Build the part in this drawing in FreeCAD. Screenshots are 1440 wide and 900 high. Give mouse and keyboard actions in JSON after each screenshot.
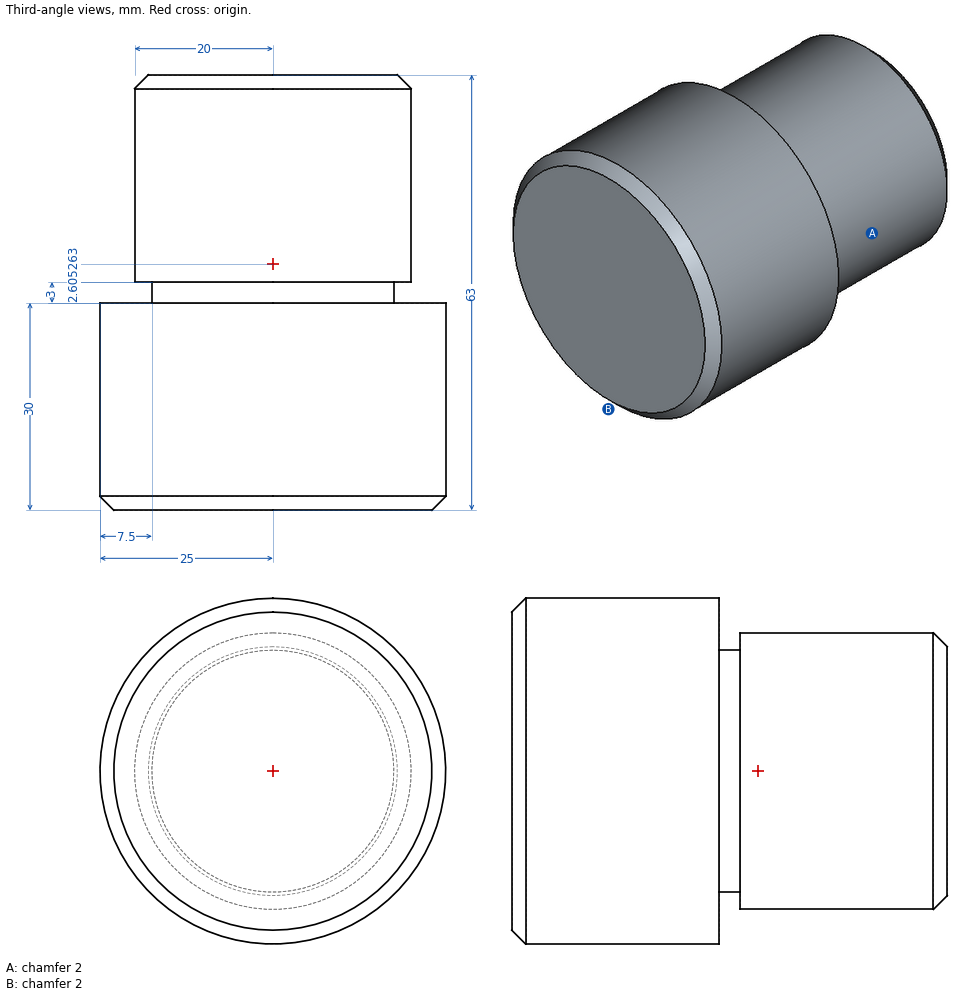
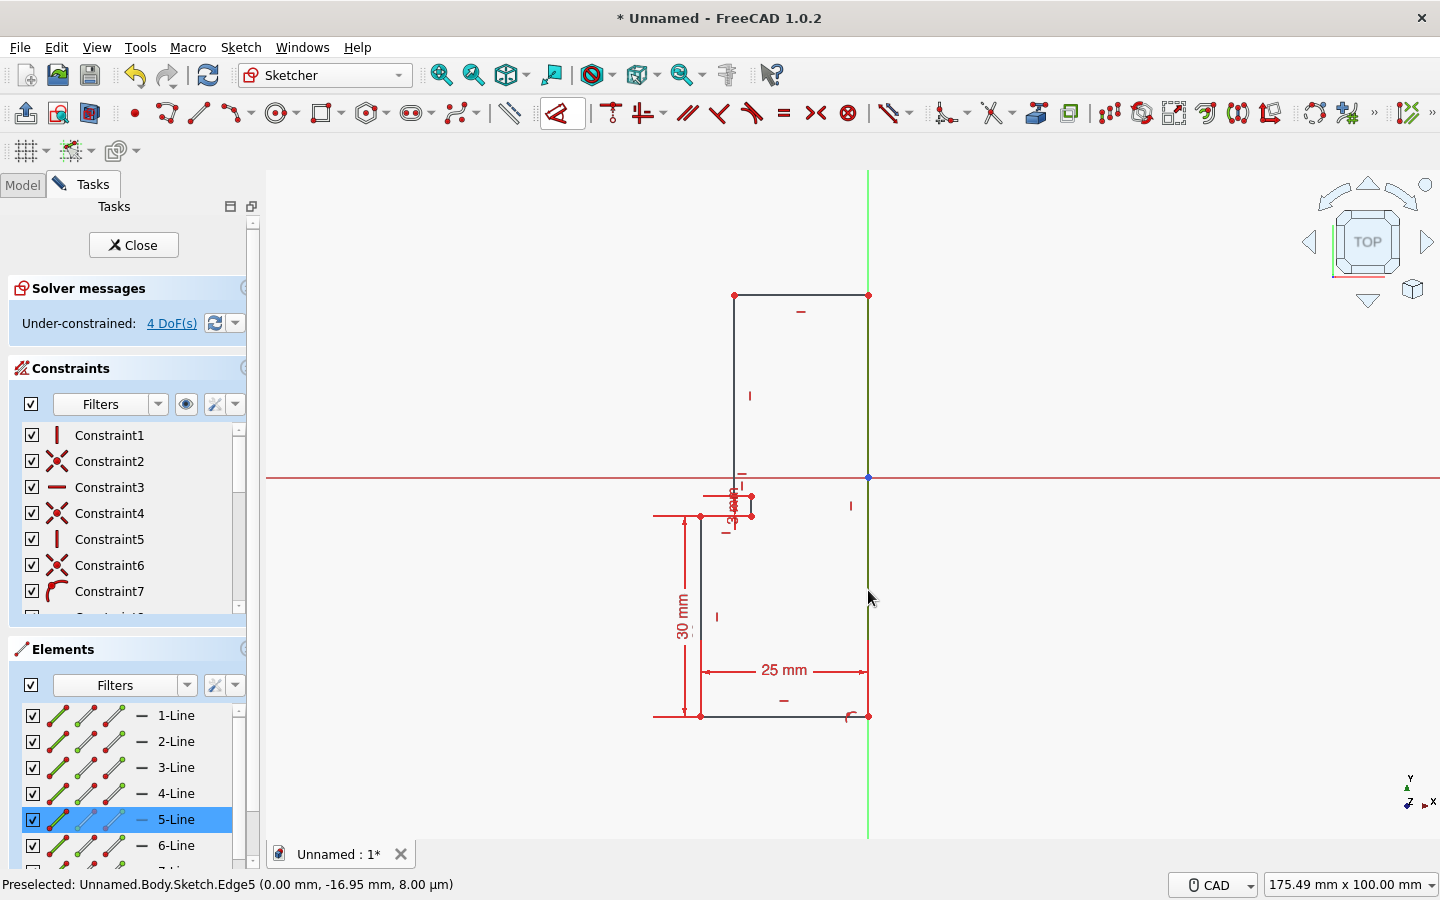
{"action": "left_click", "coordinate": [580, 114]}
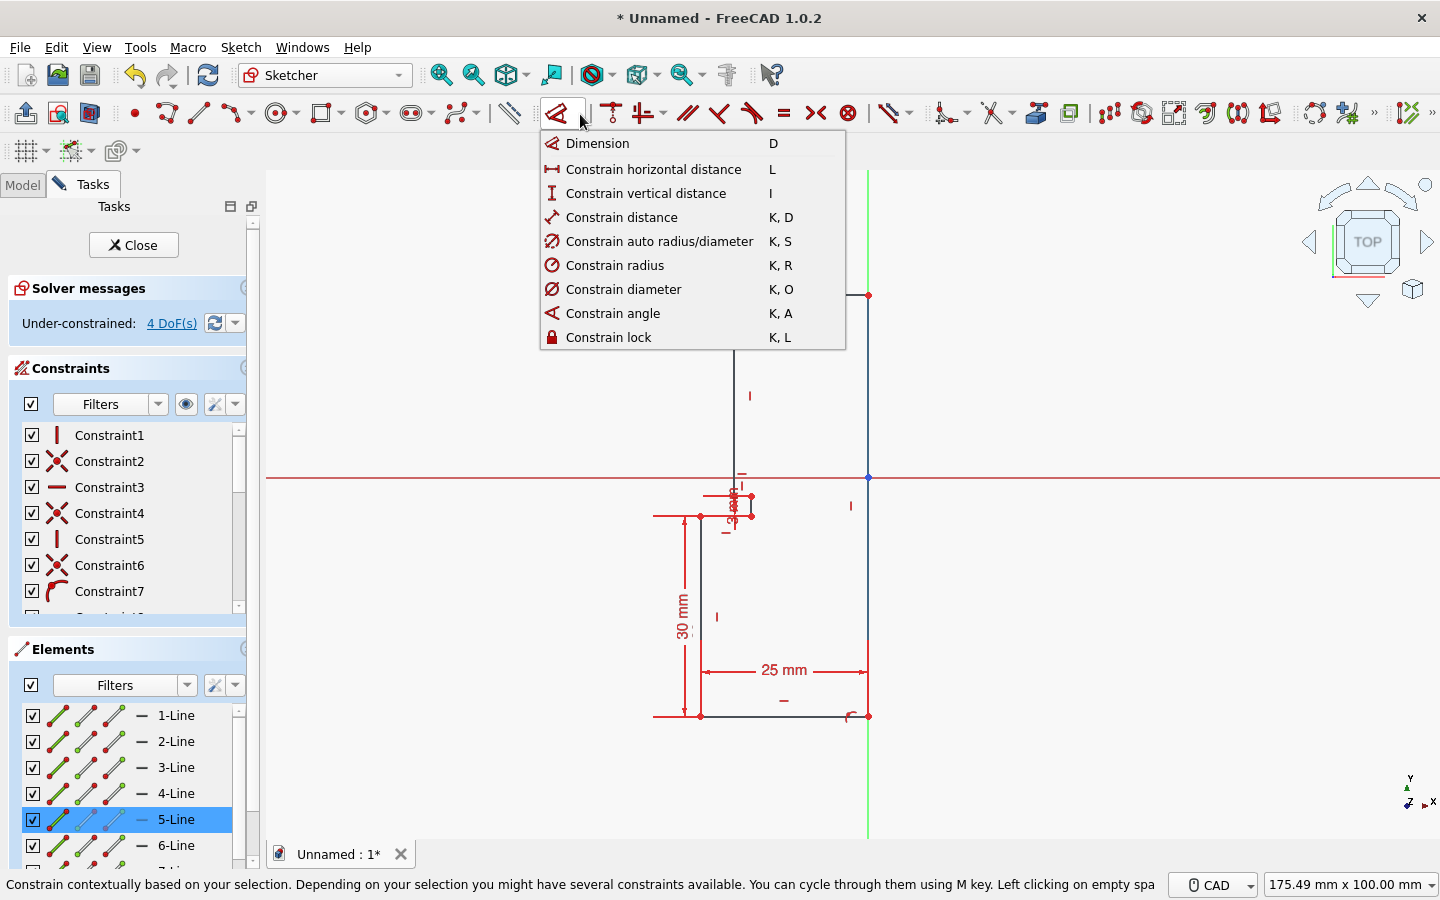
{"action": "left_click", "coordinate": [693, 193]}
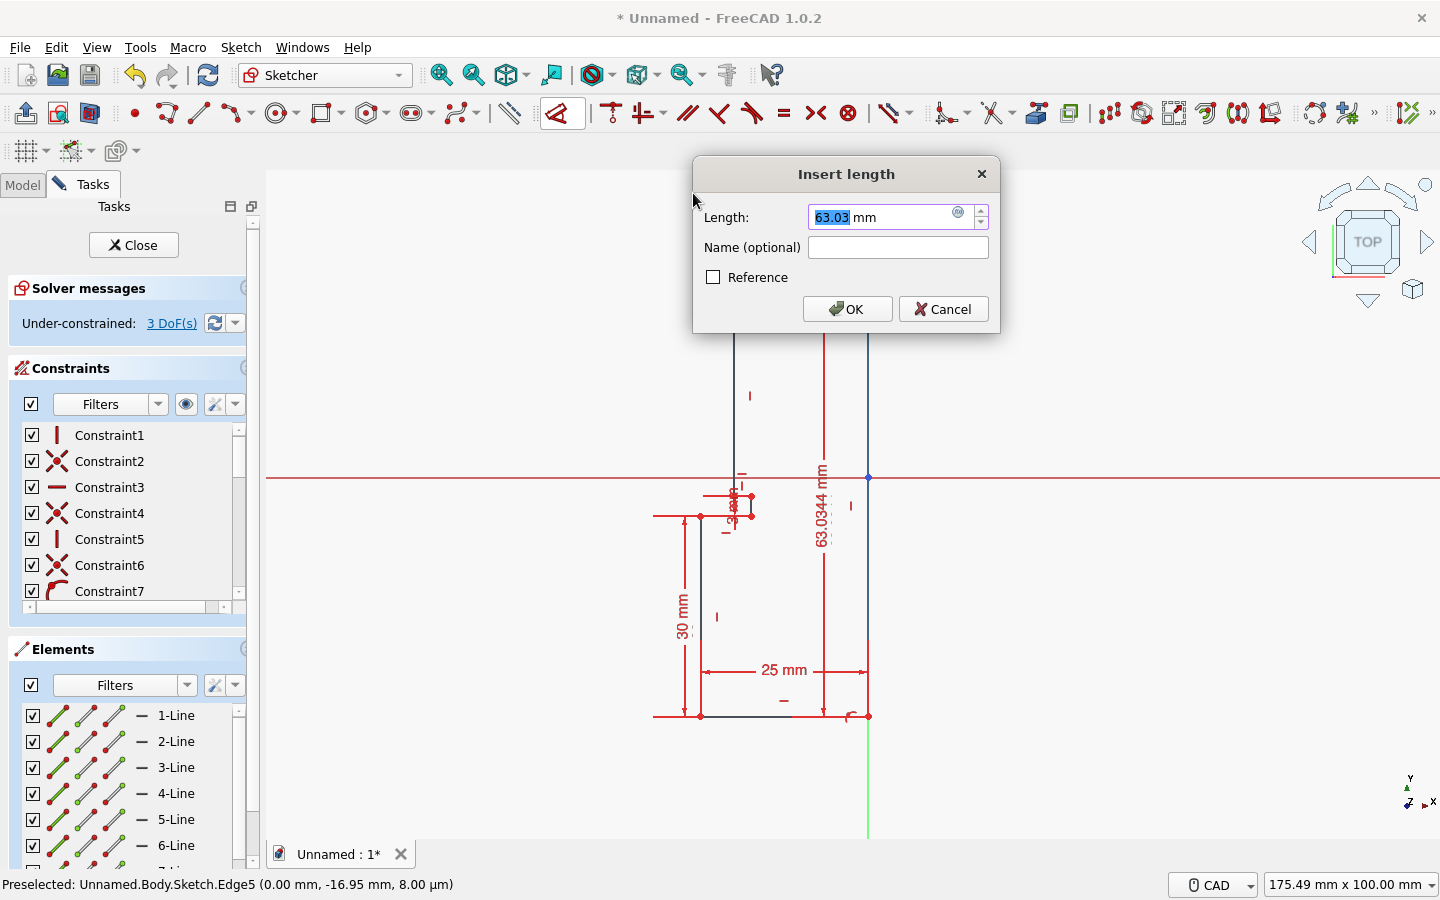
{"action": "type", "text": "63"}
{"action": "key", "text": "Return"}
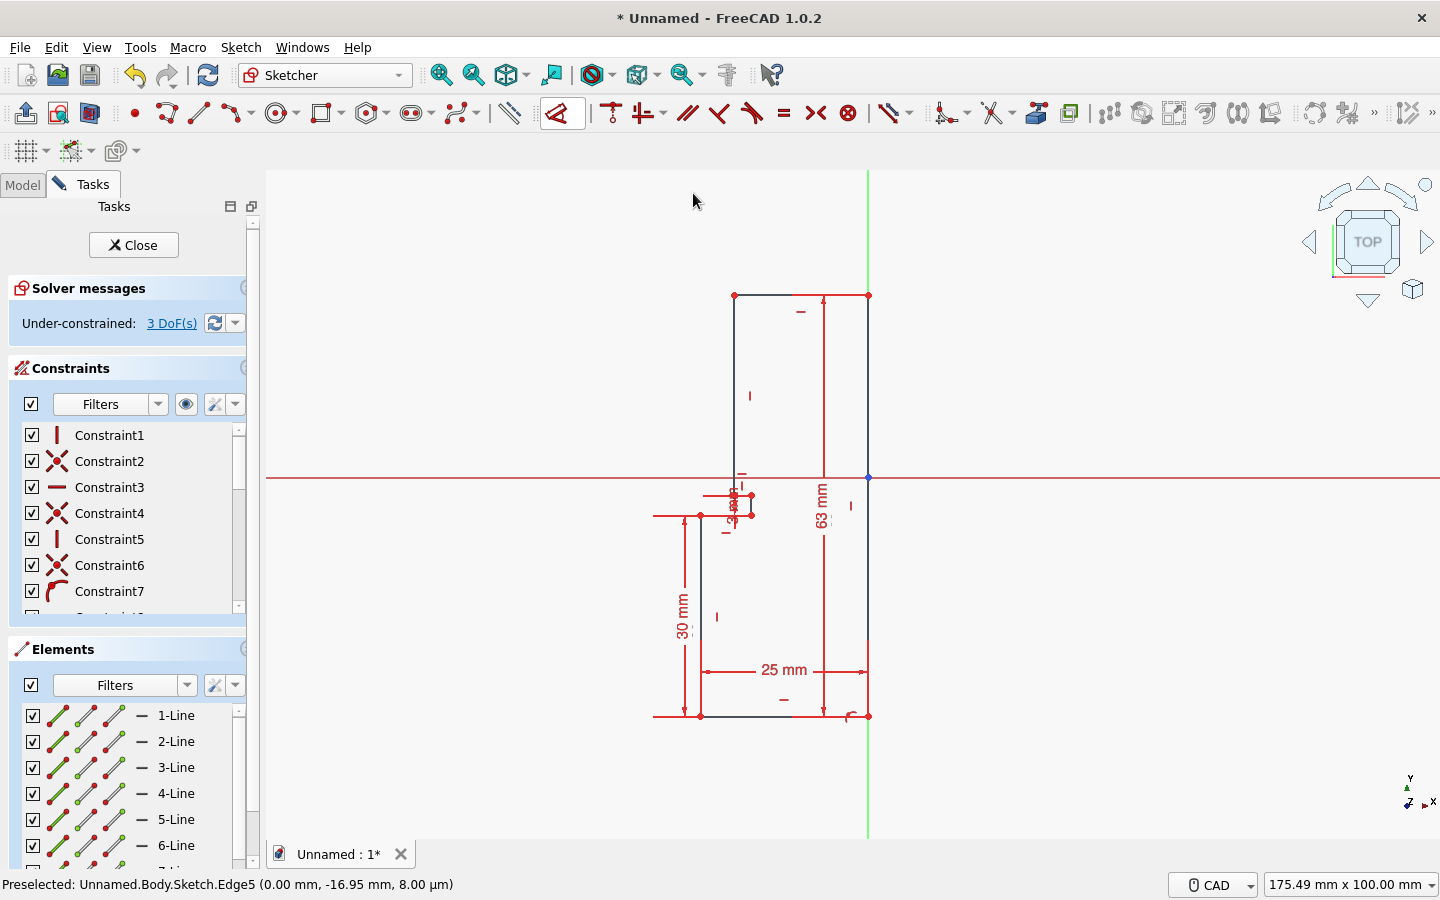
{"action": "left_click", "coordinate": [828, 295]}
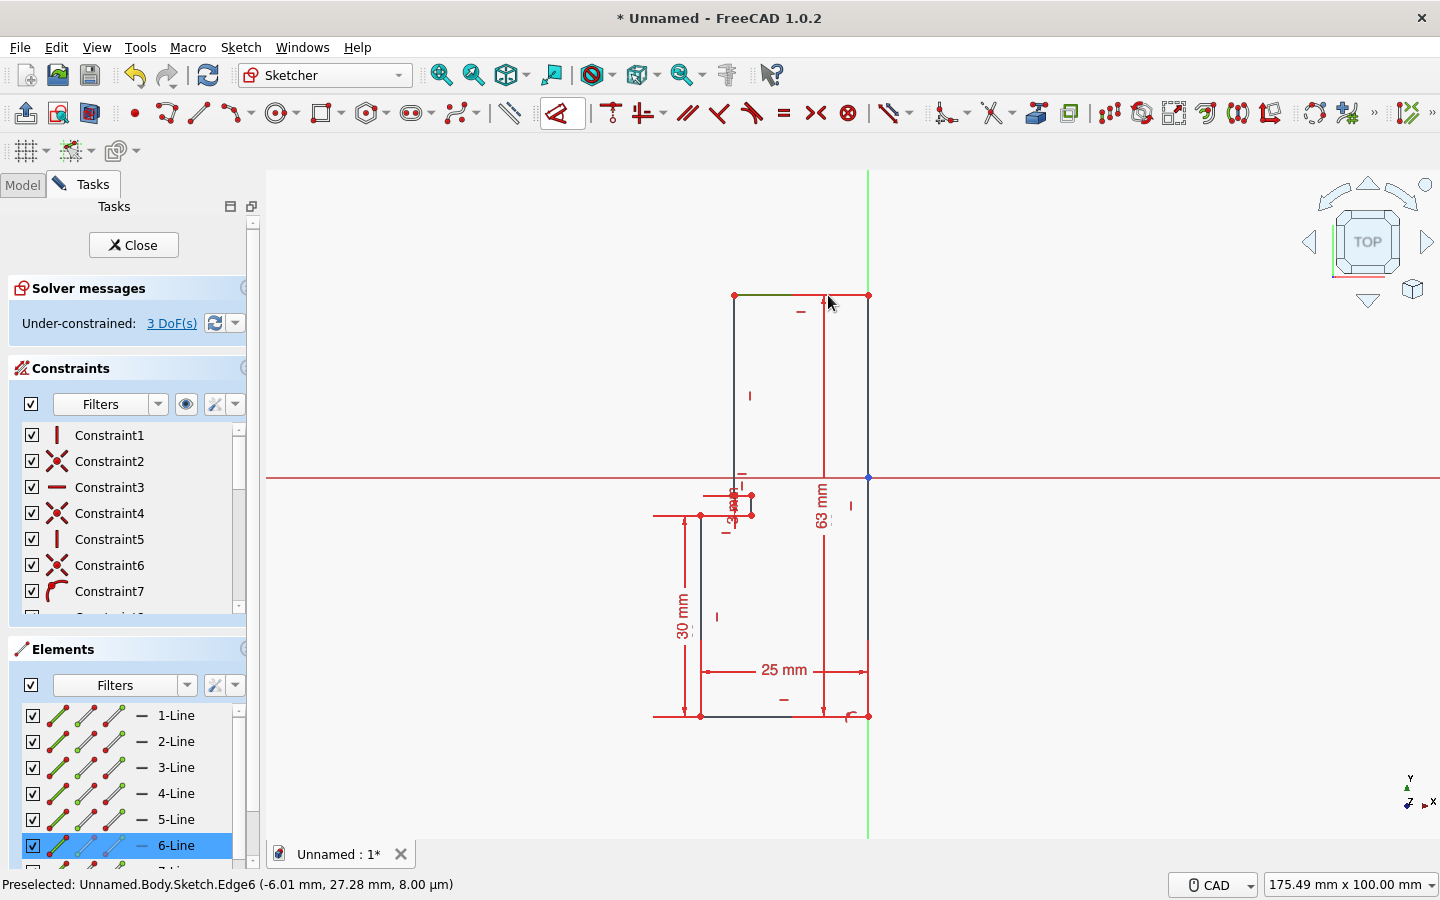
{"action": "left_click", "coordinate": [580, 114]}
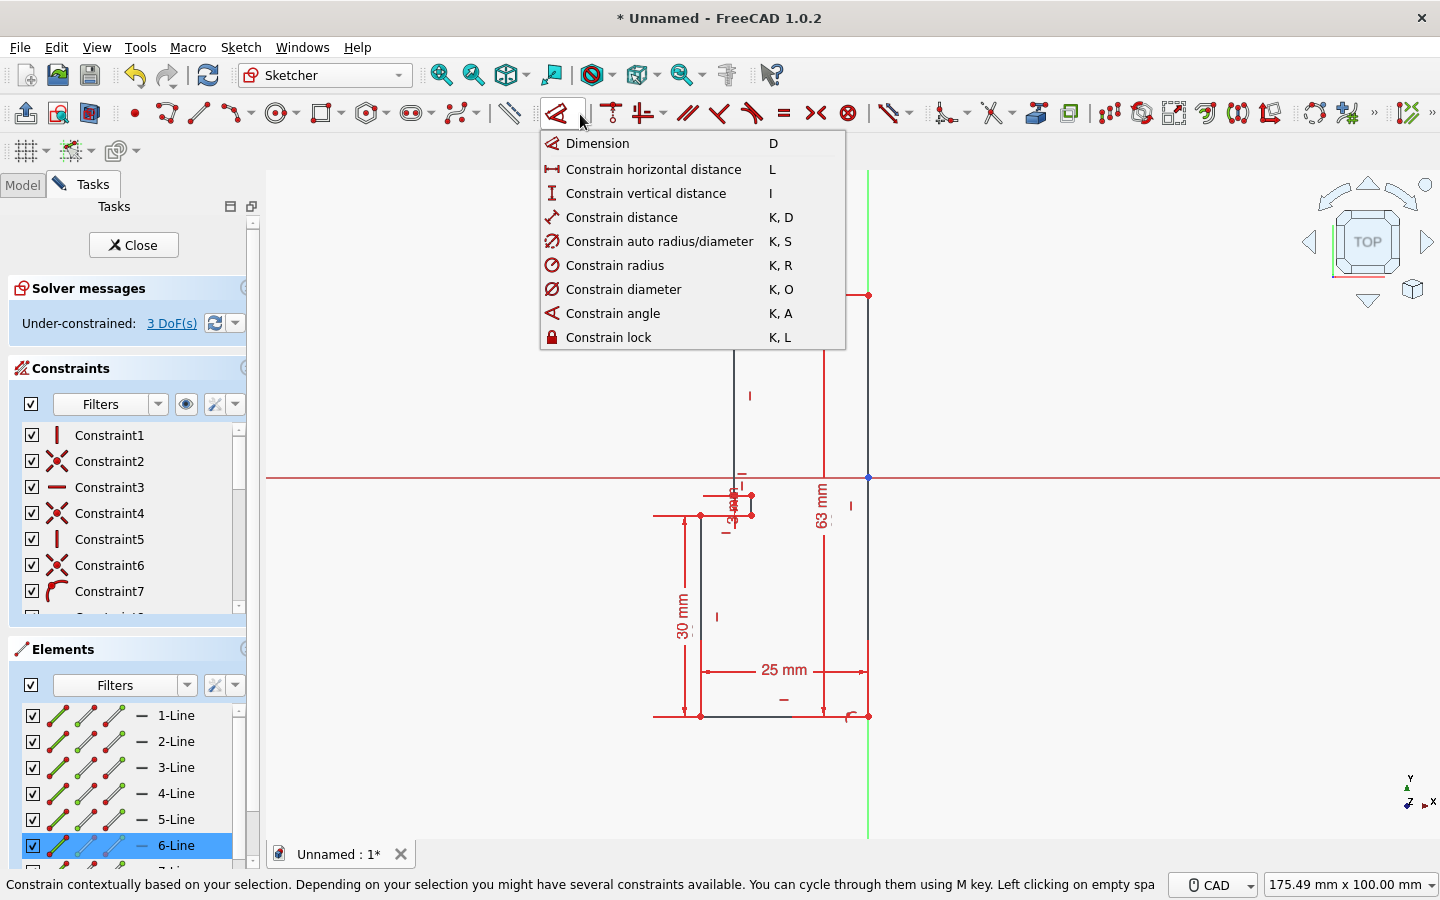
{"action": "left_click", "coordinate": [693, 169]}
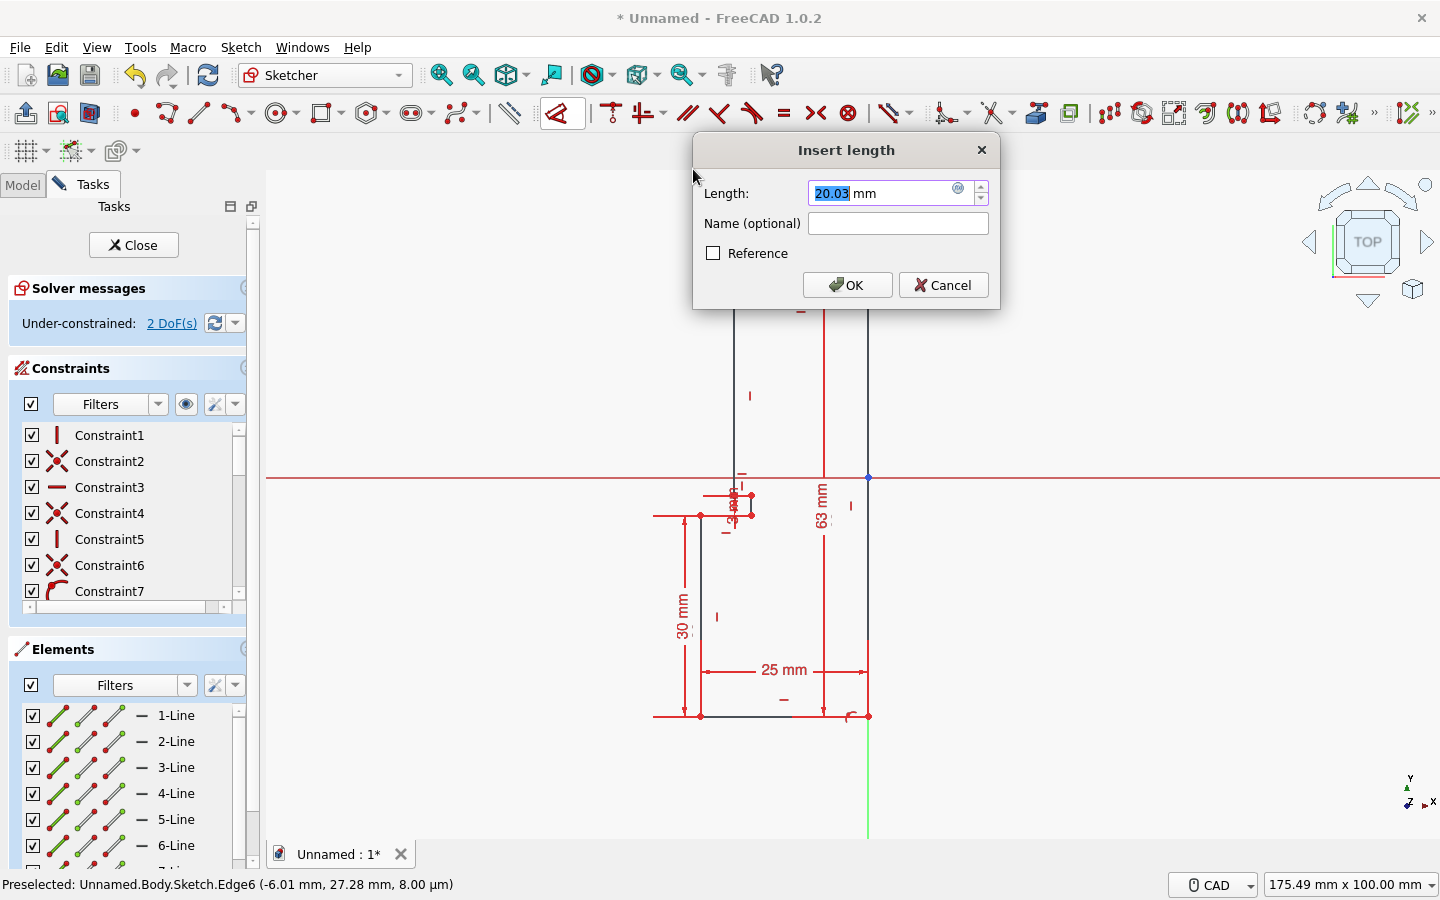
{"action": "type", "text": "20"}
{"action": "key", "text": "Return"}